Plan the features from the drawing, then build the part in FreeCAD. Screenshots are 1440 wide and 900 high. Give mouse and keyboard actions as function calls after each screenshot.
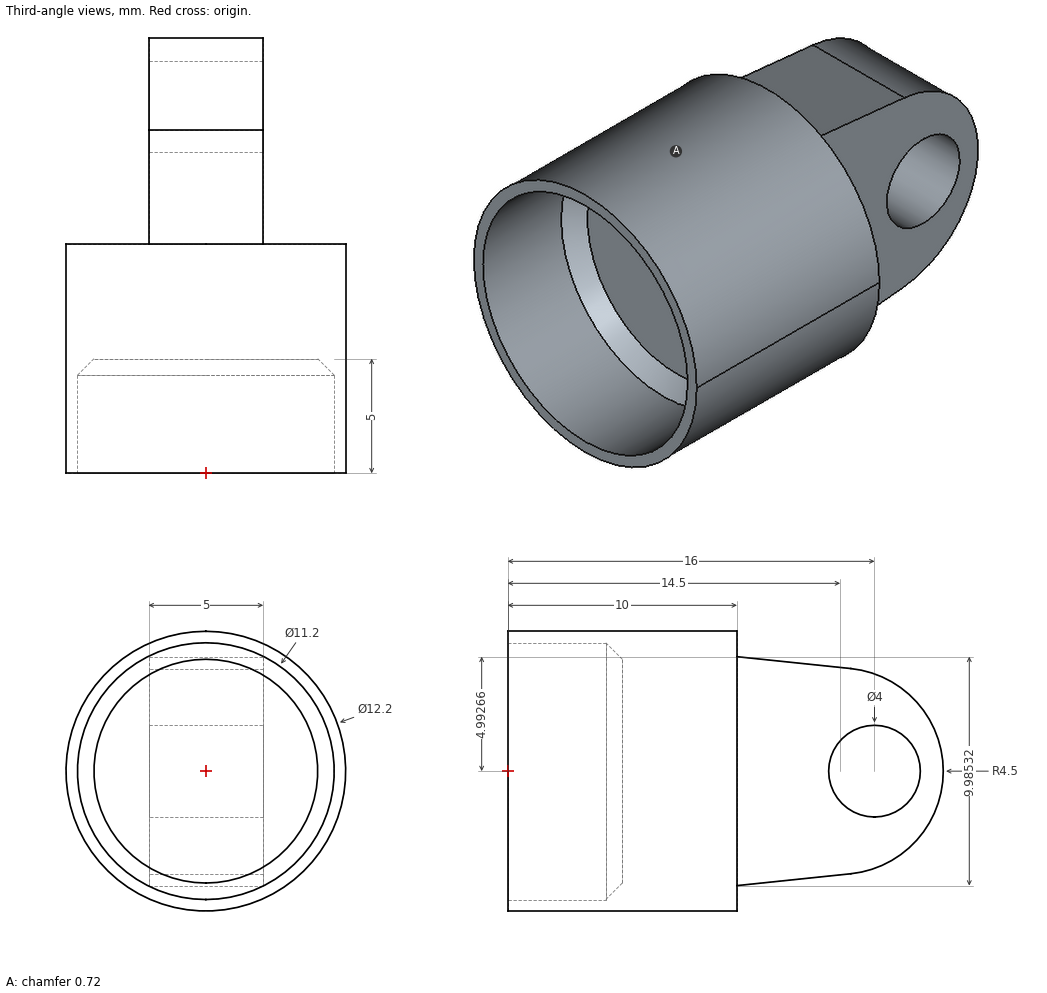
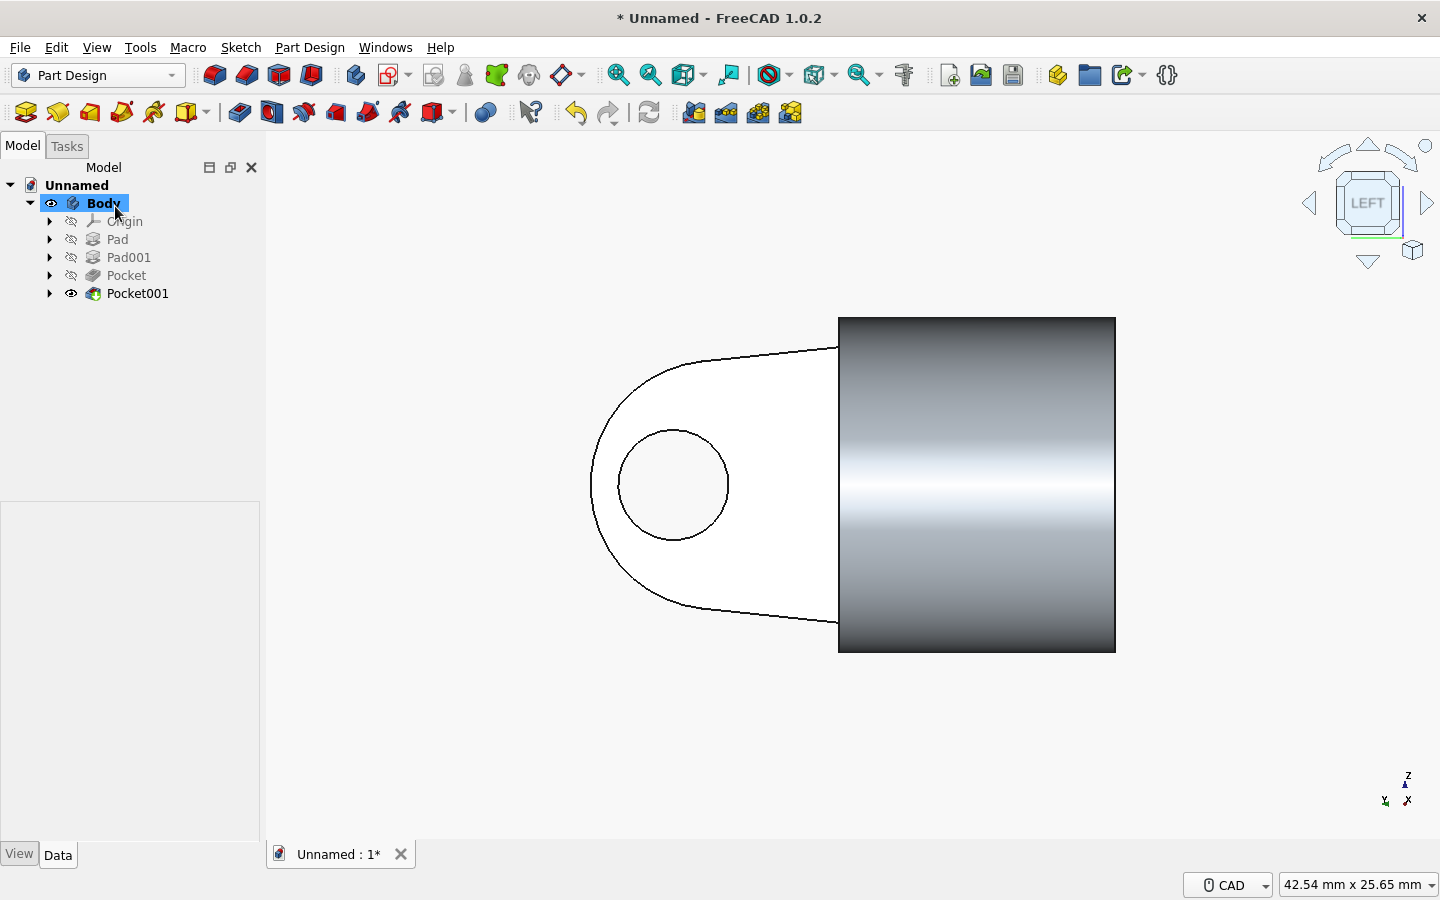
key(v)
key(3)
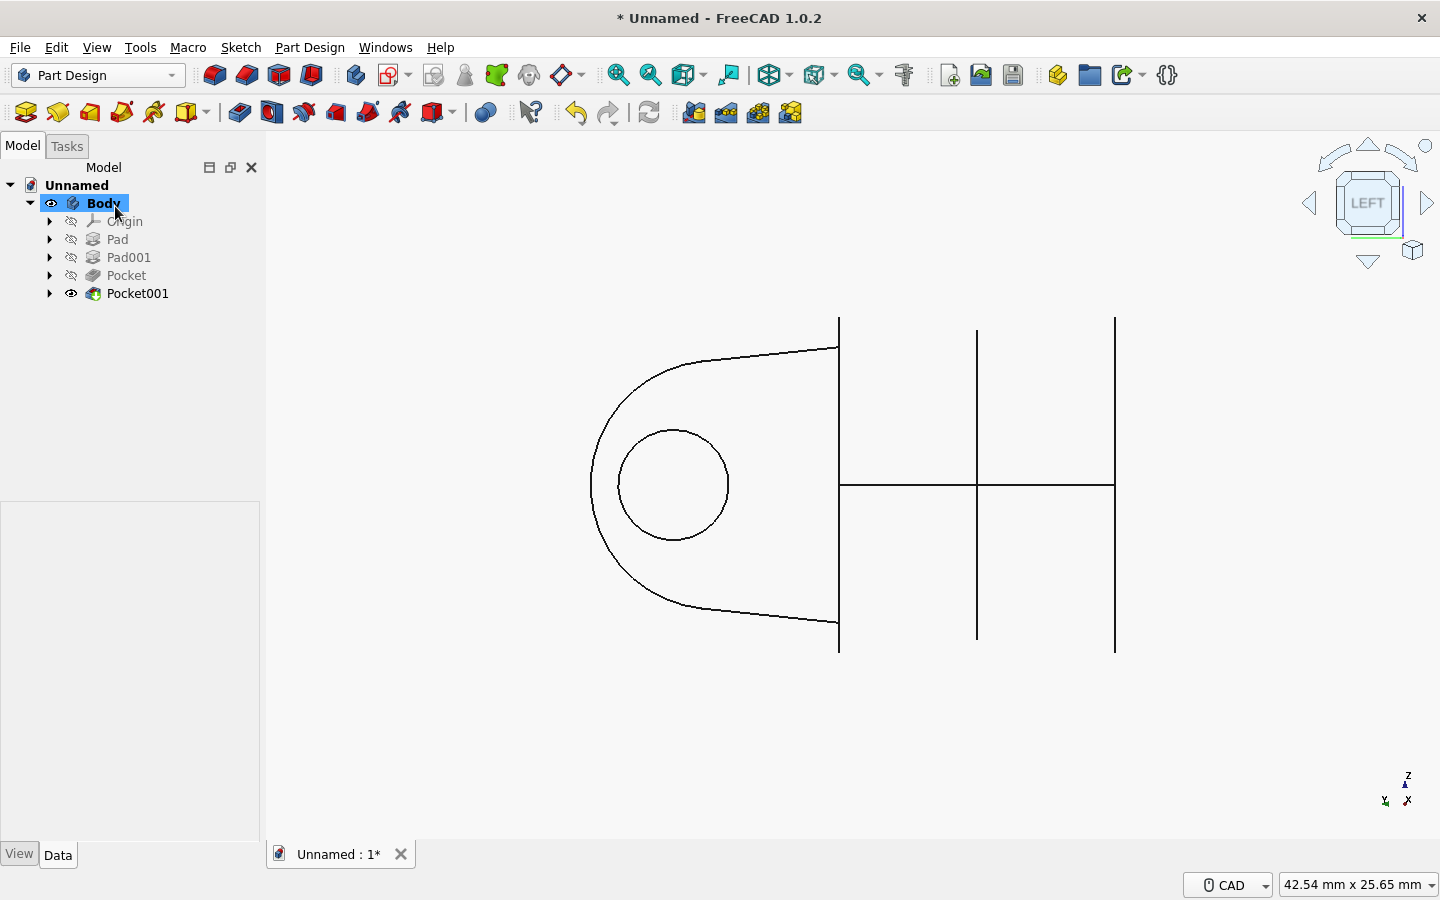
key(0)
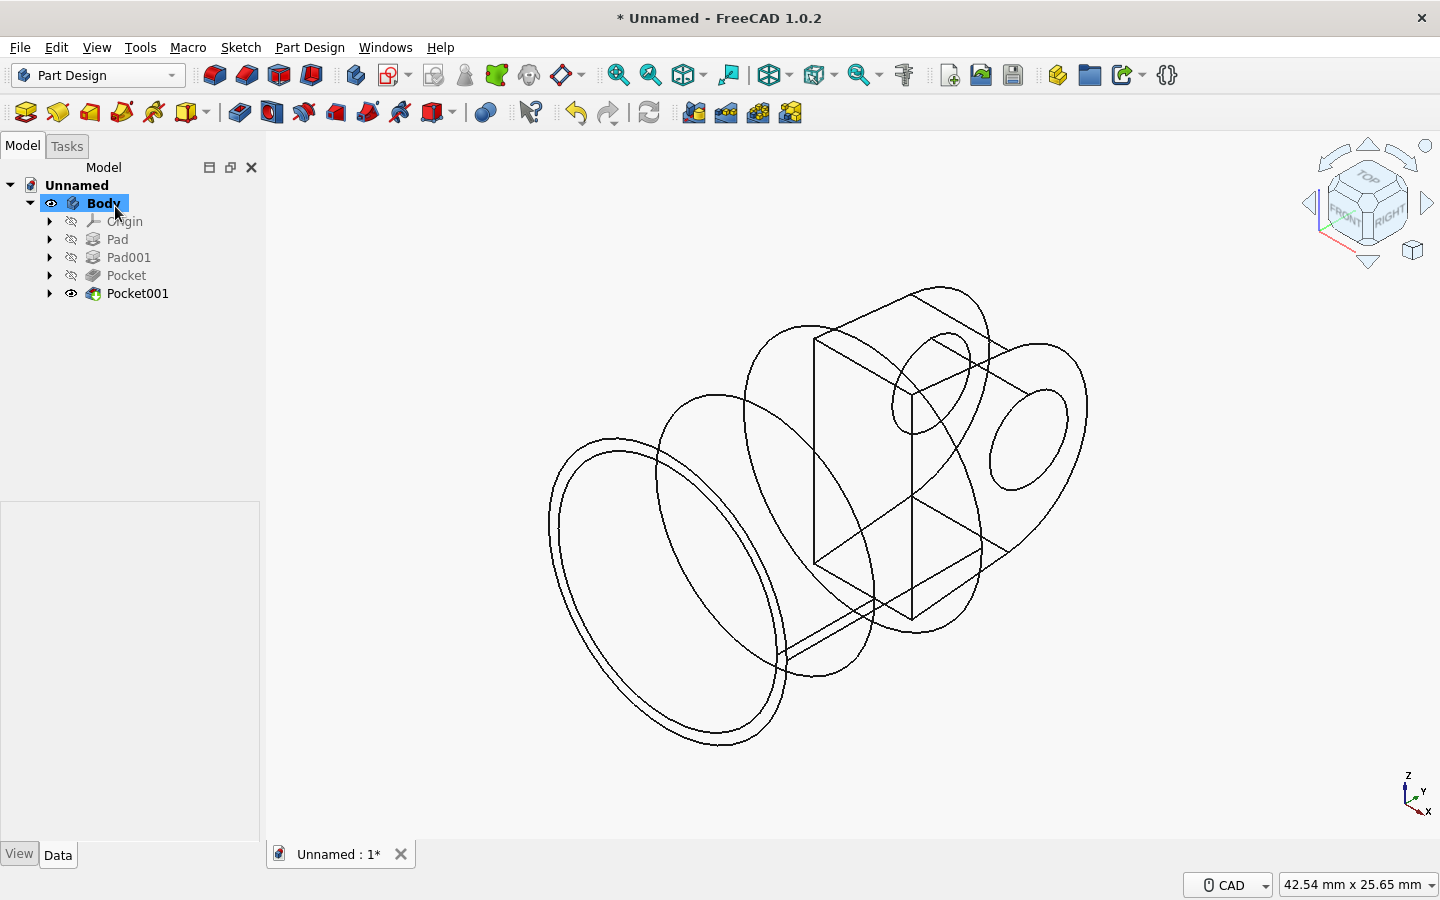
click(656, 472)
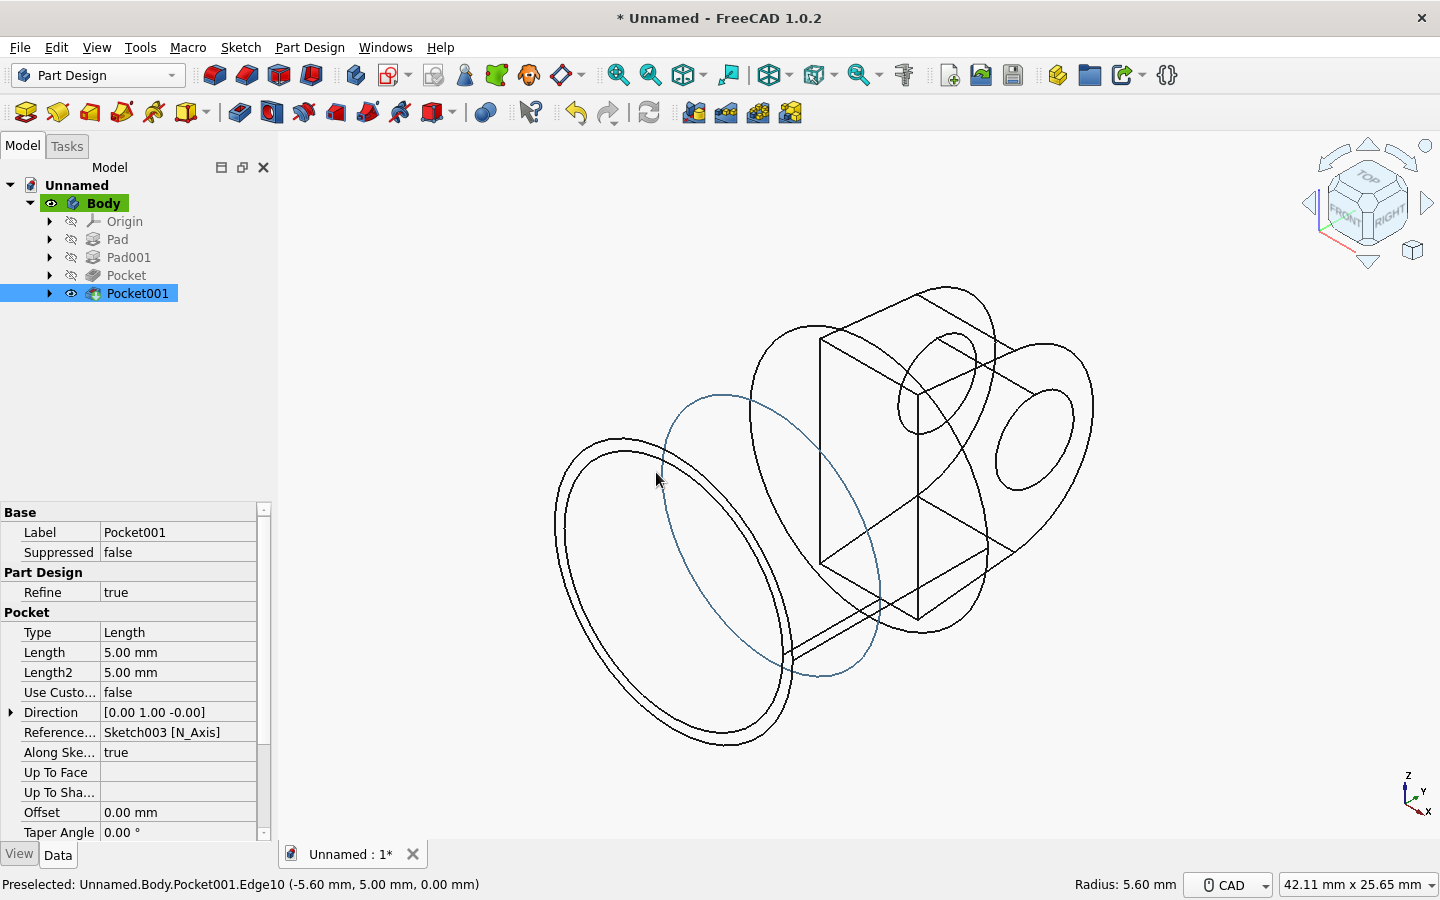
key(v)
key(1)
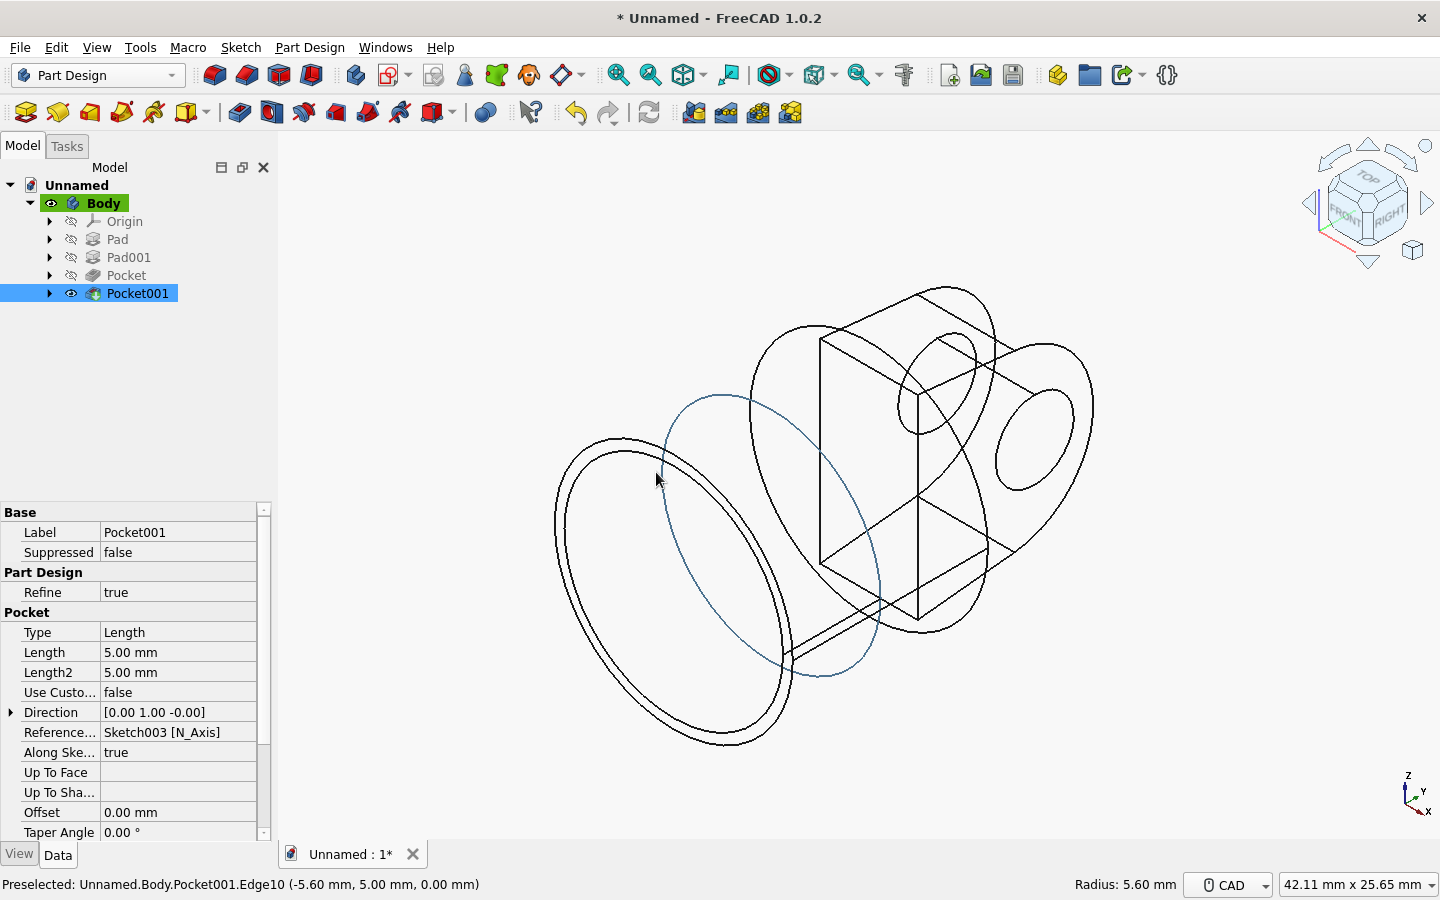
click(248, 76)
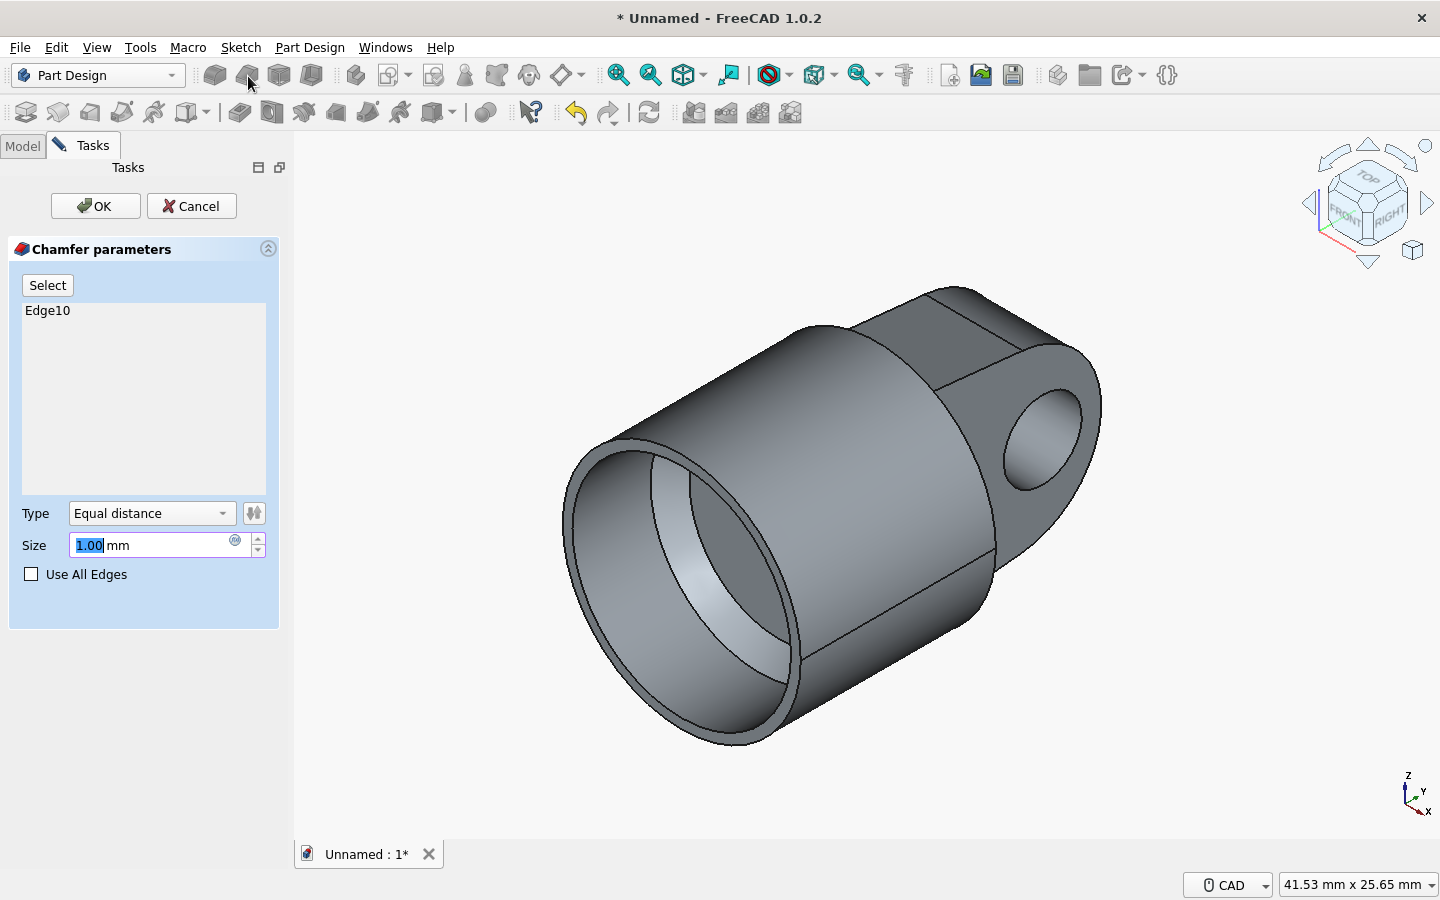
text(0.72)
key(Tab)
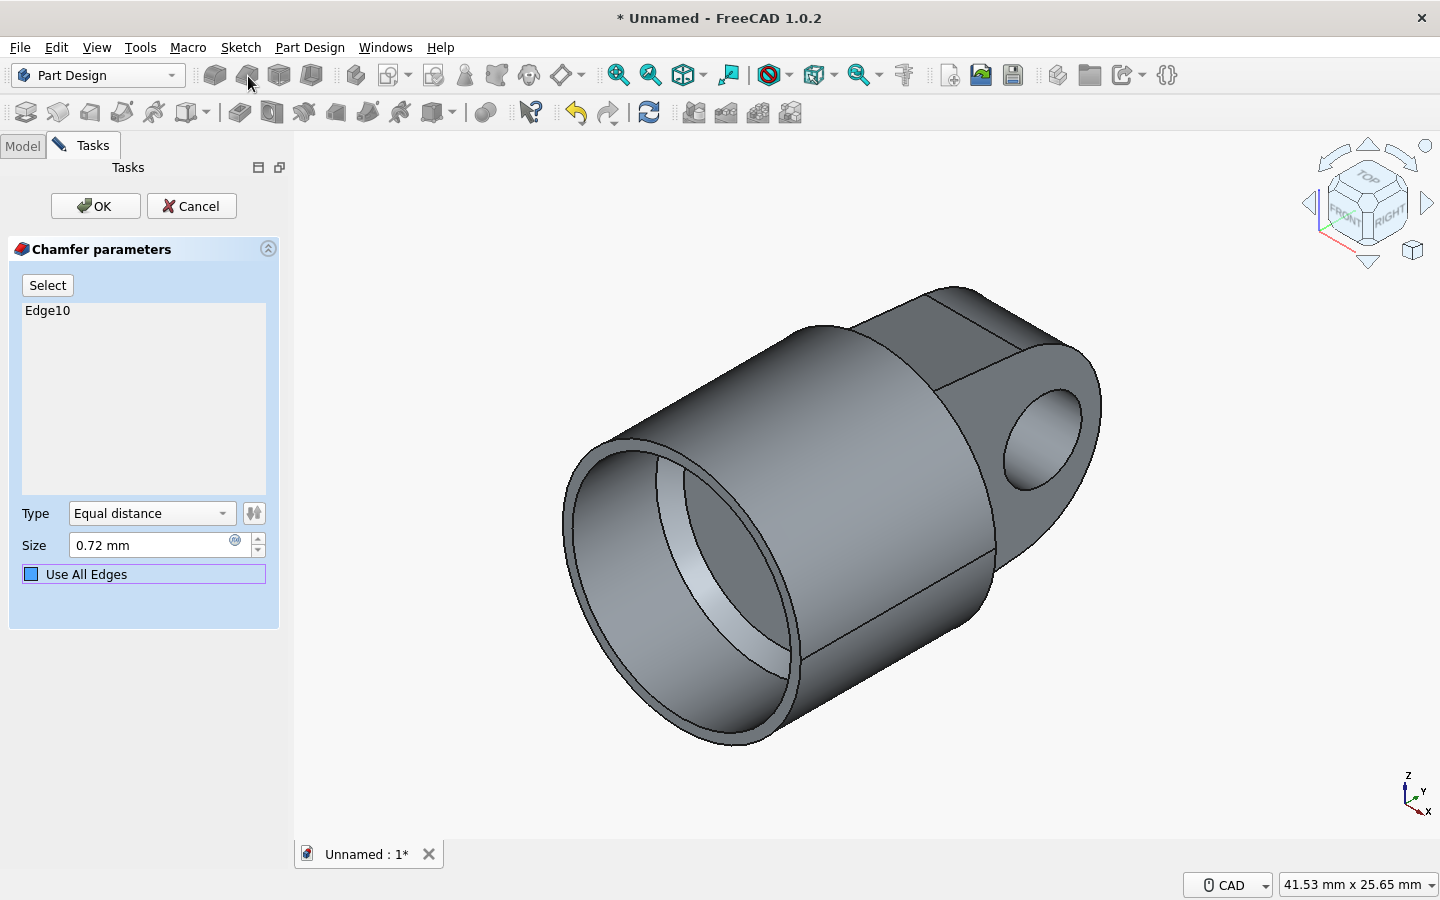
click(96, 206)